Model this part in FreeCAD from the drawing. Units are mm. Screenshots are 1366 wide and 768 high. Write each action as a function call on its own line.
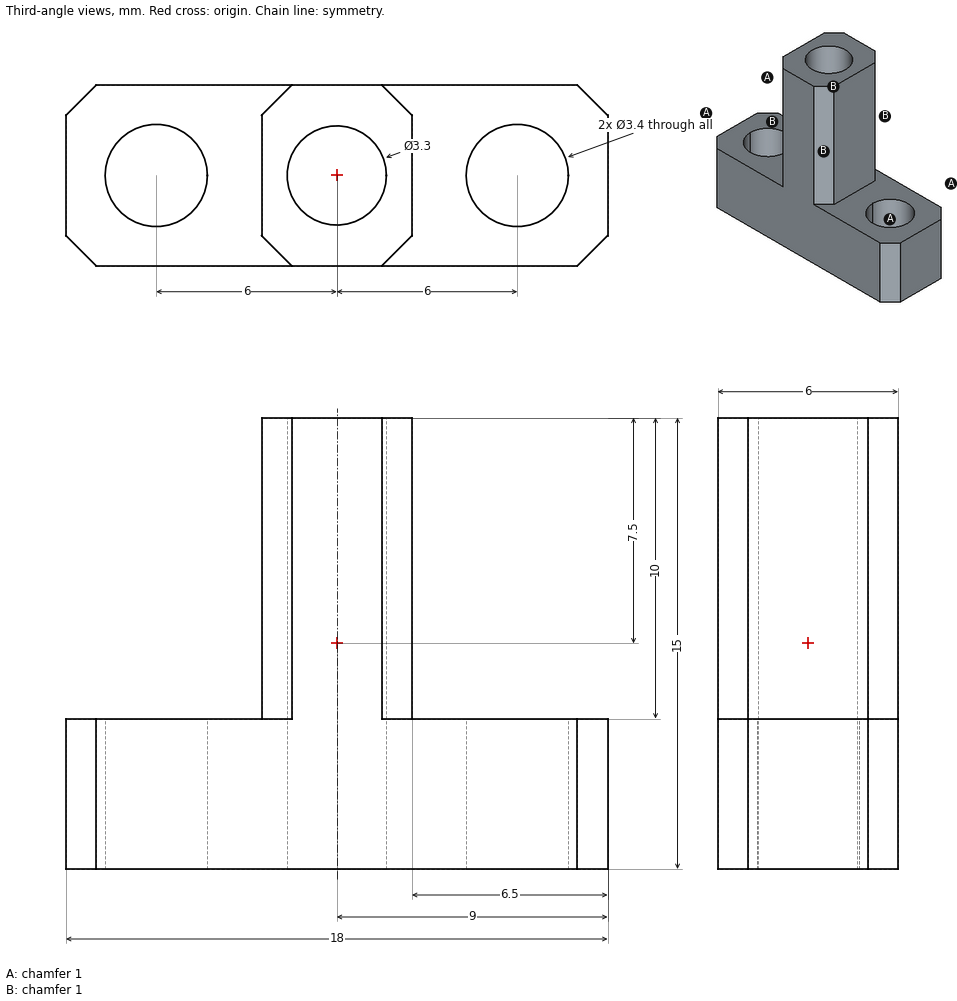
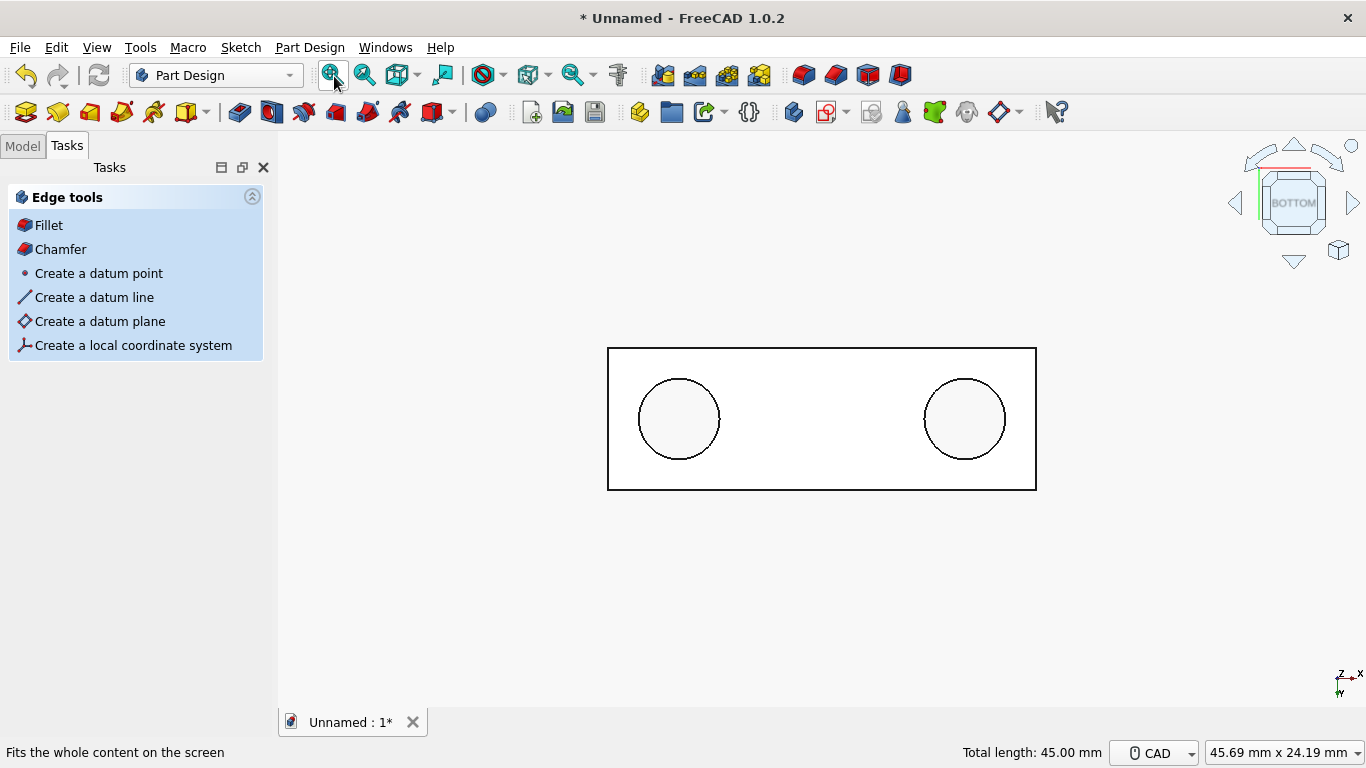
key(4)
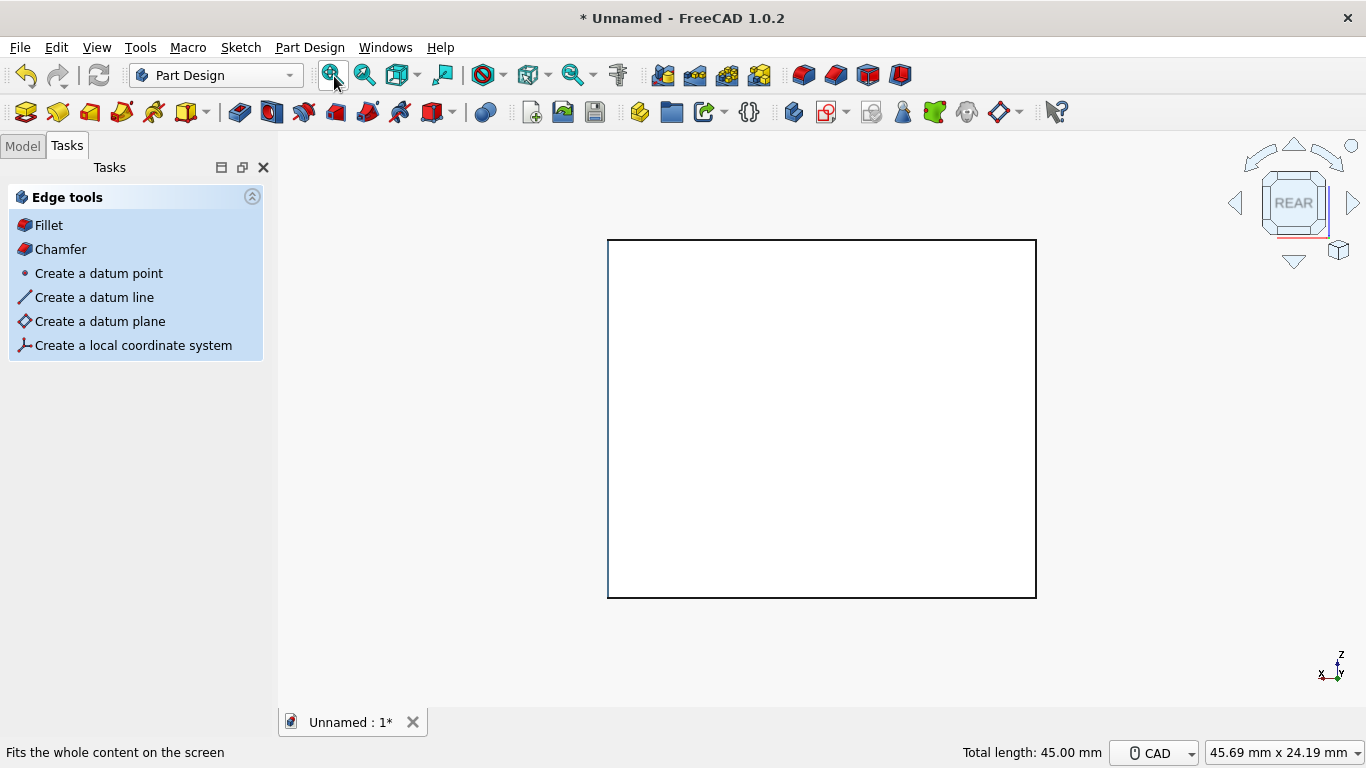
click(1036, 418, ctrl)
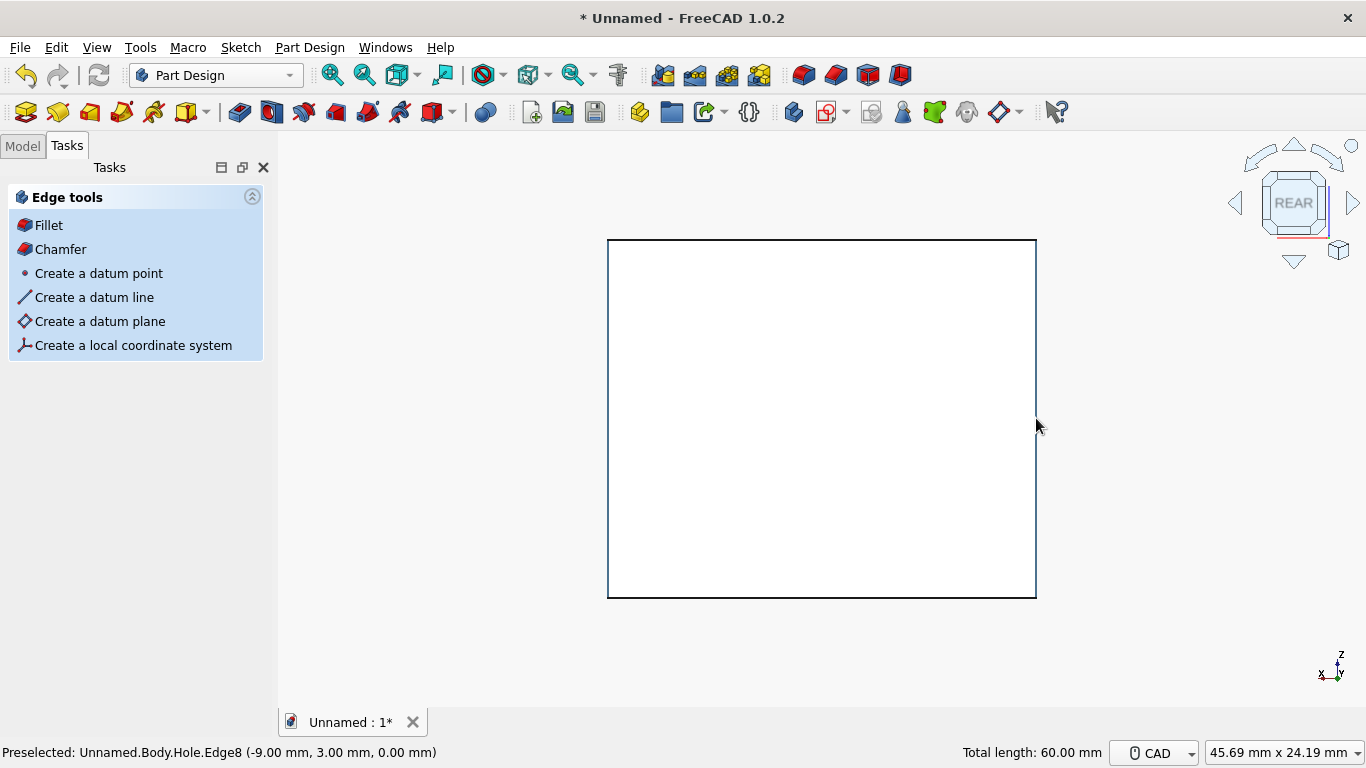
click(836, 76)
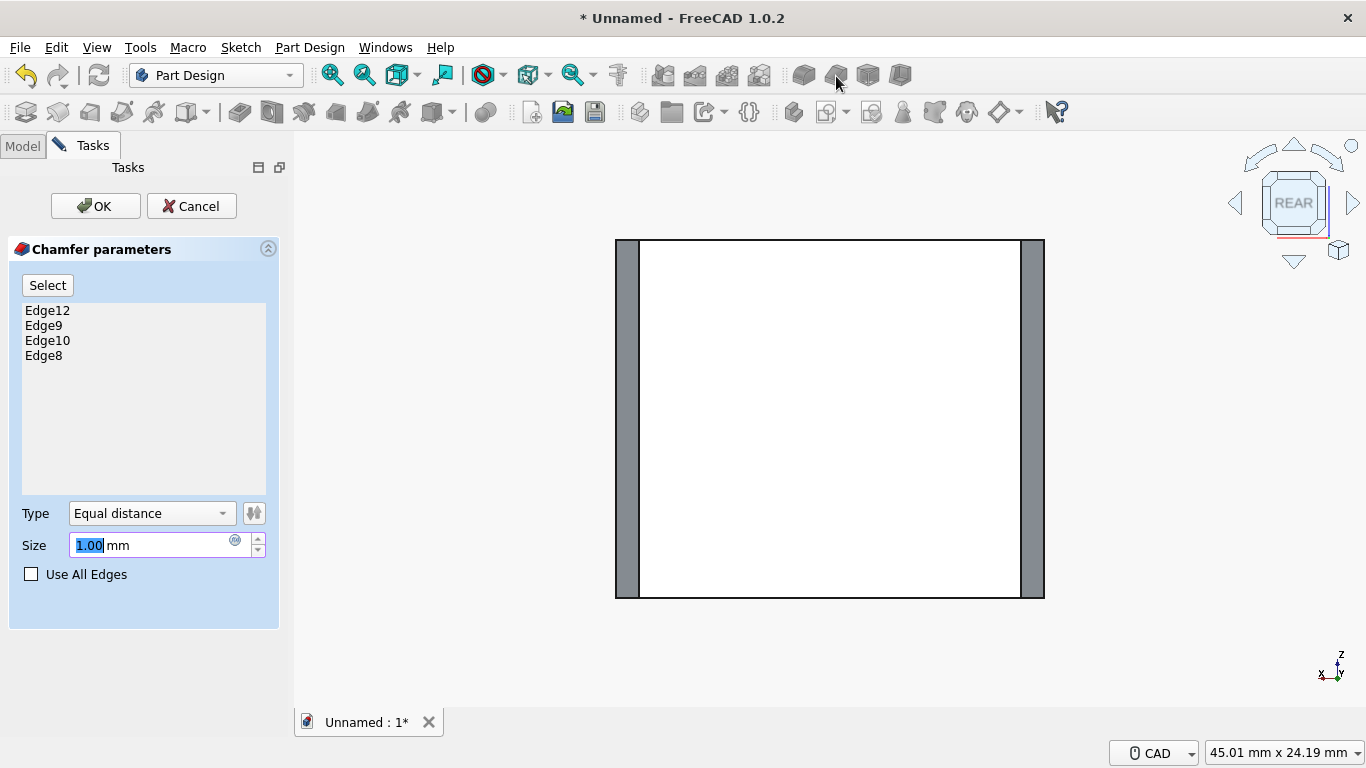
text(1)
key(Tab)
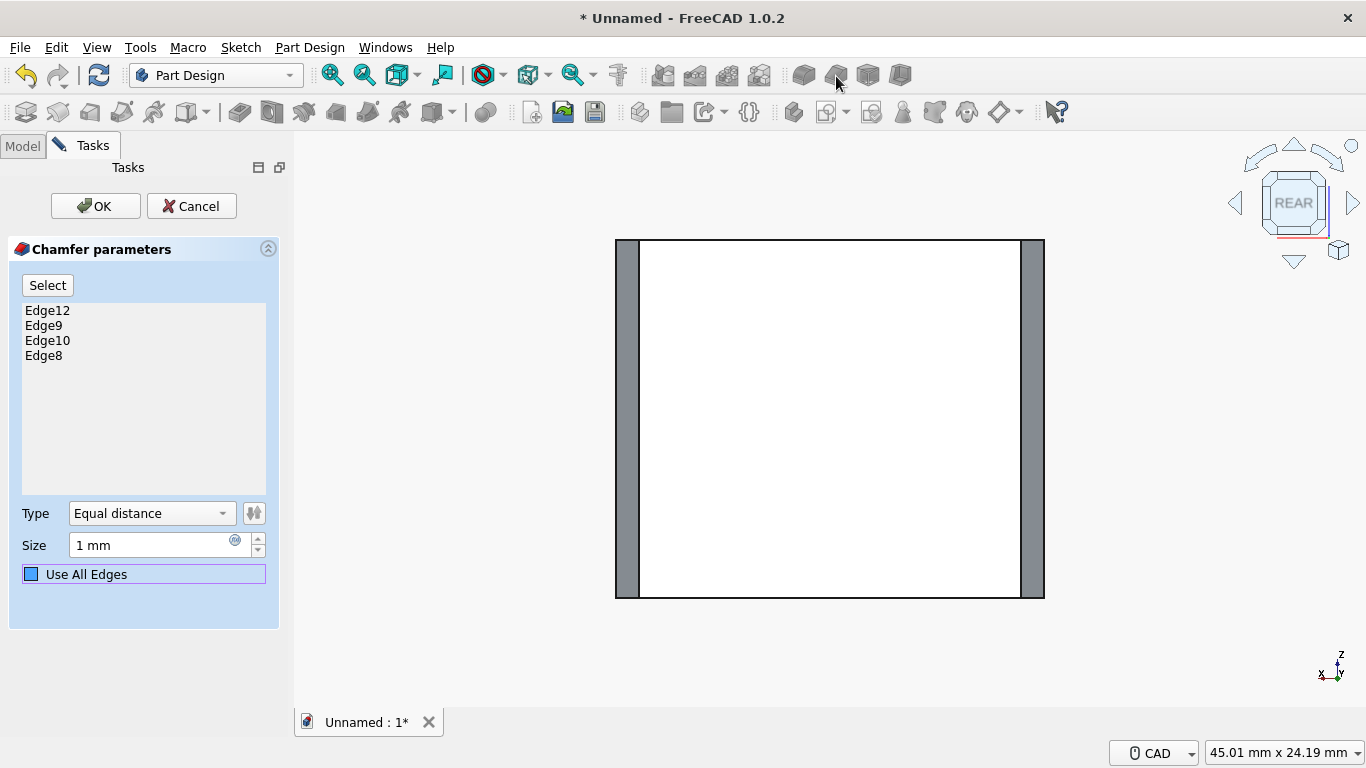
click(96, 206)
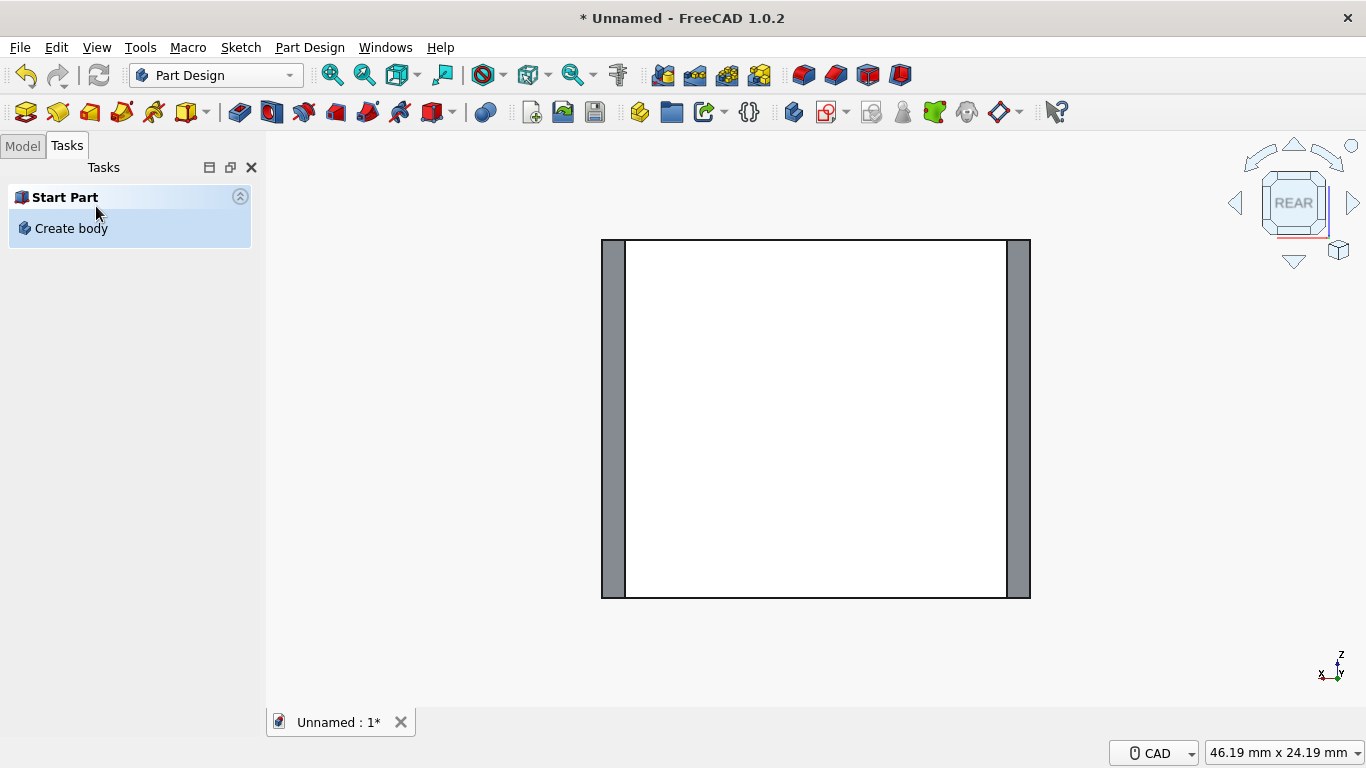
key(0)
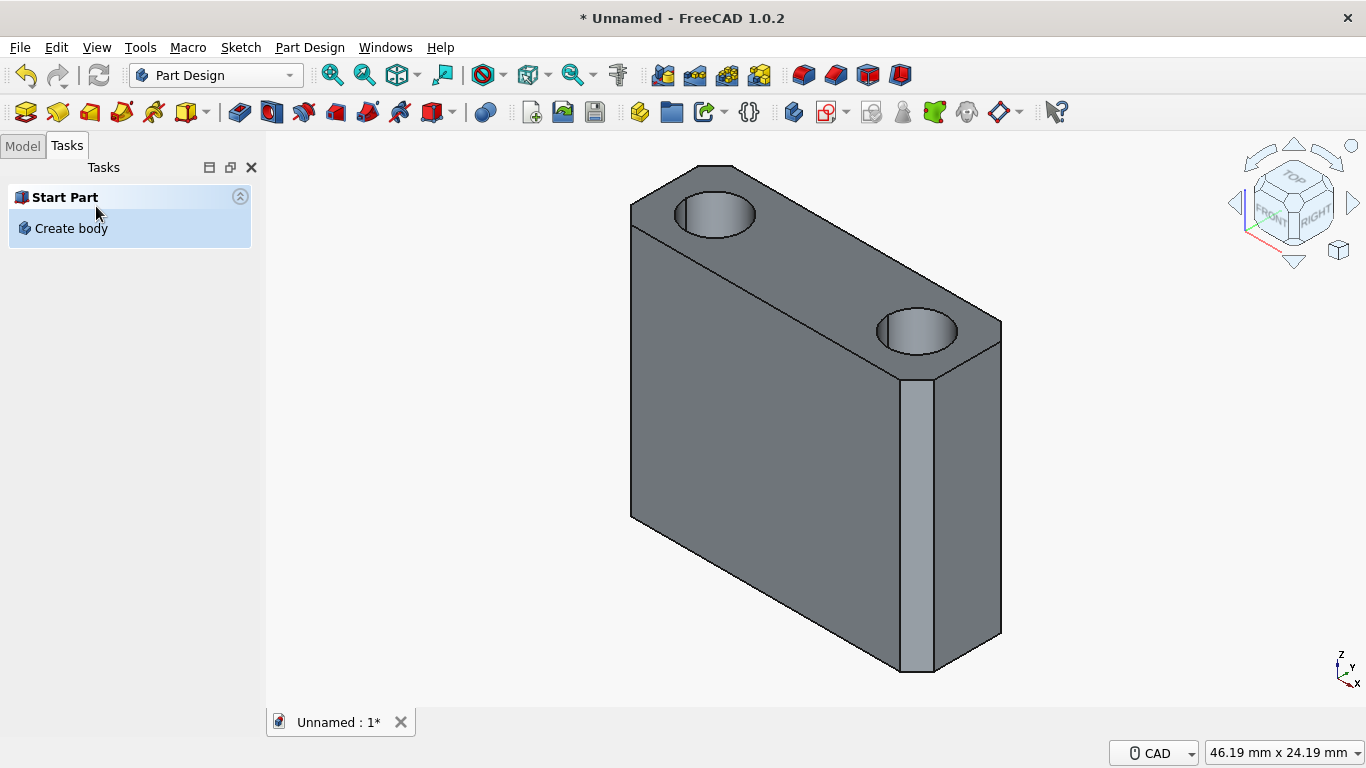
click(765, 447)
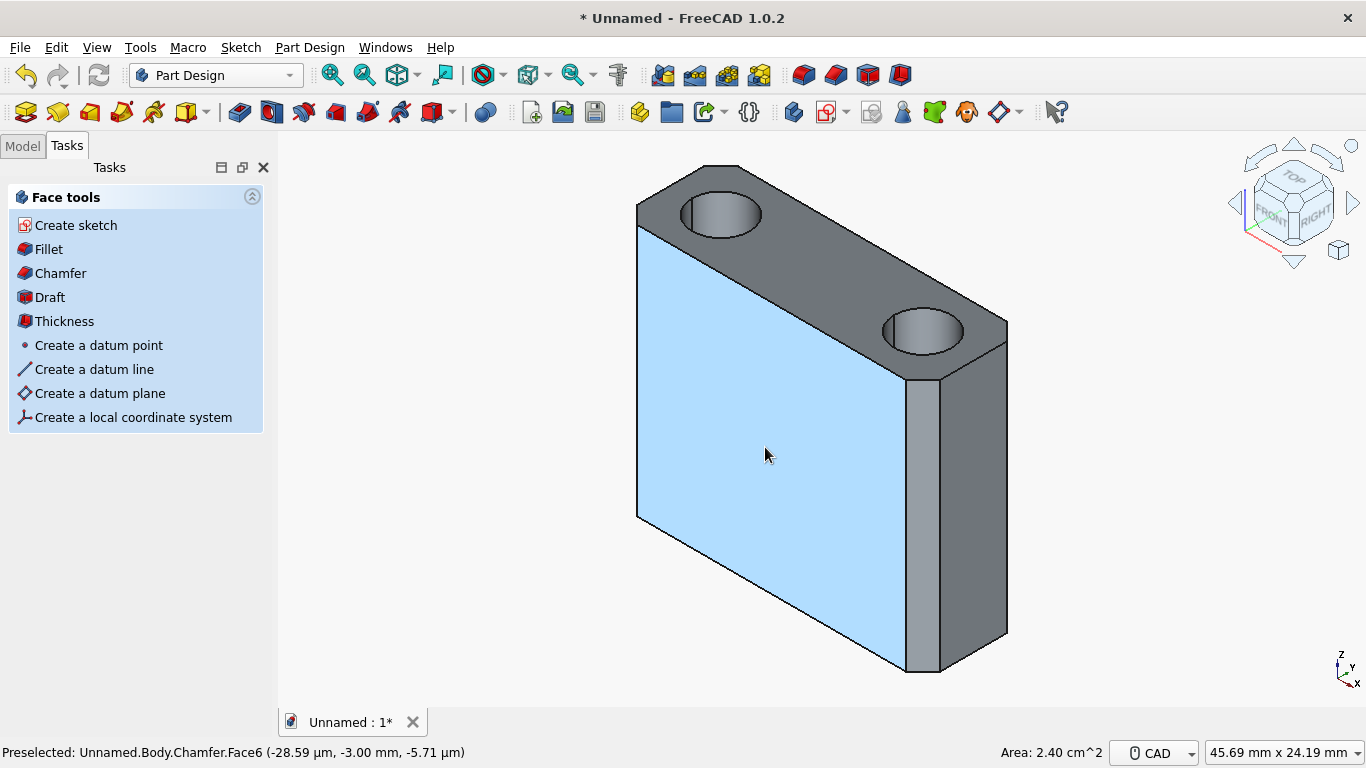
click(826, 112)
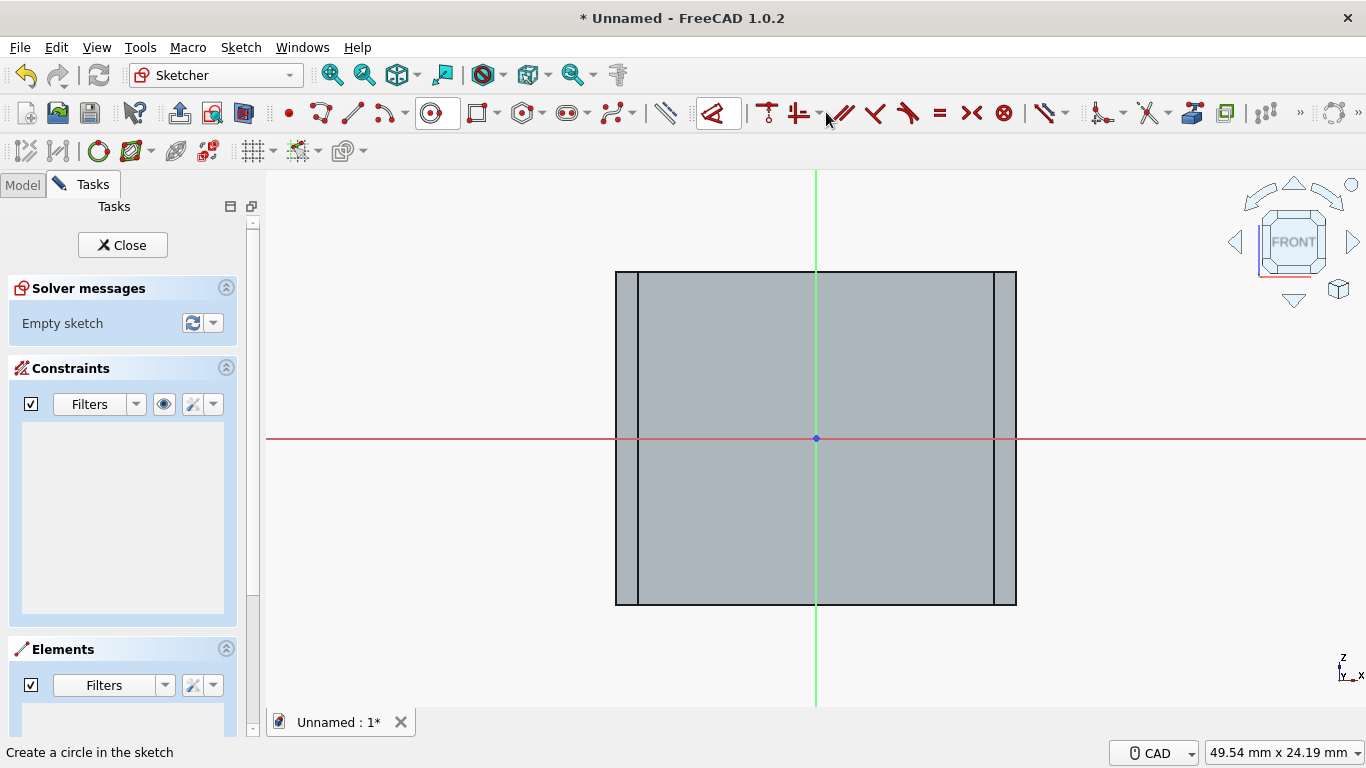
scroll(955, 270, up, 2)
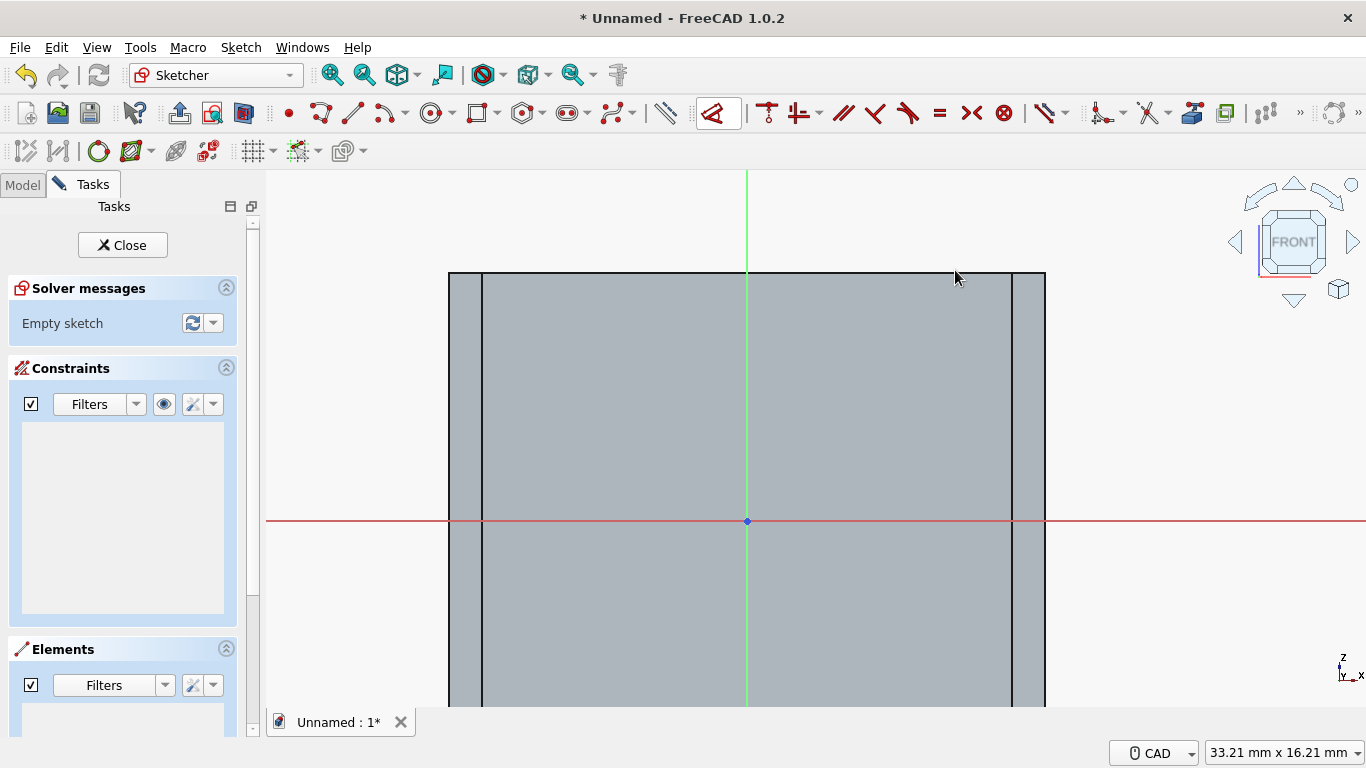
click(478, 114)